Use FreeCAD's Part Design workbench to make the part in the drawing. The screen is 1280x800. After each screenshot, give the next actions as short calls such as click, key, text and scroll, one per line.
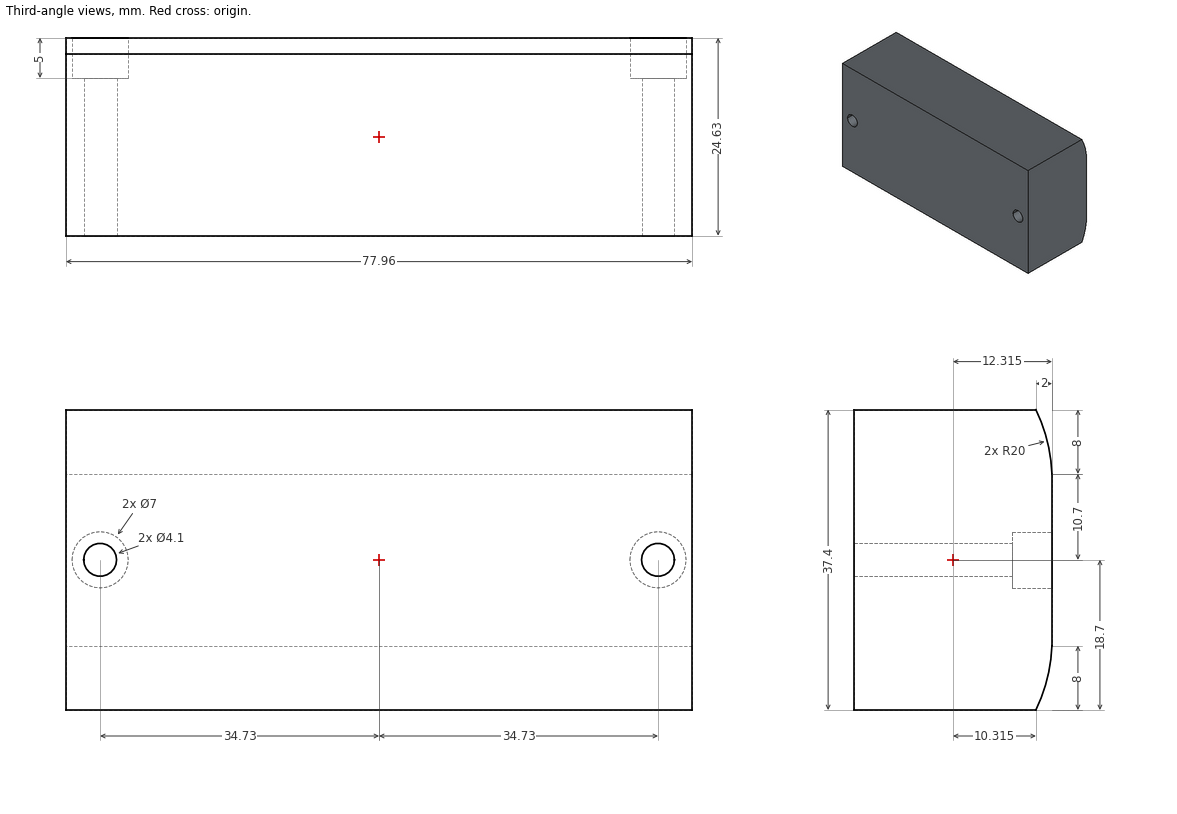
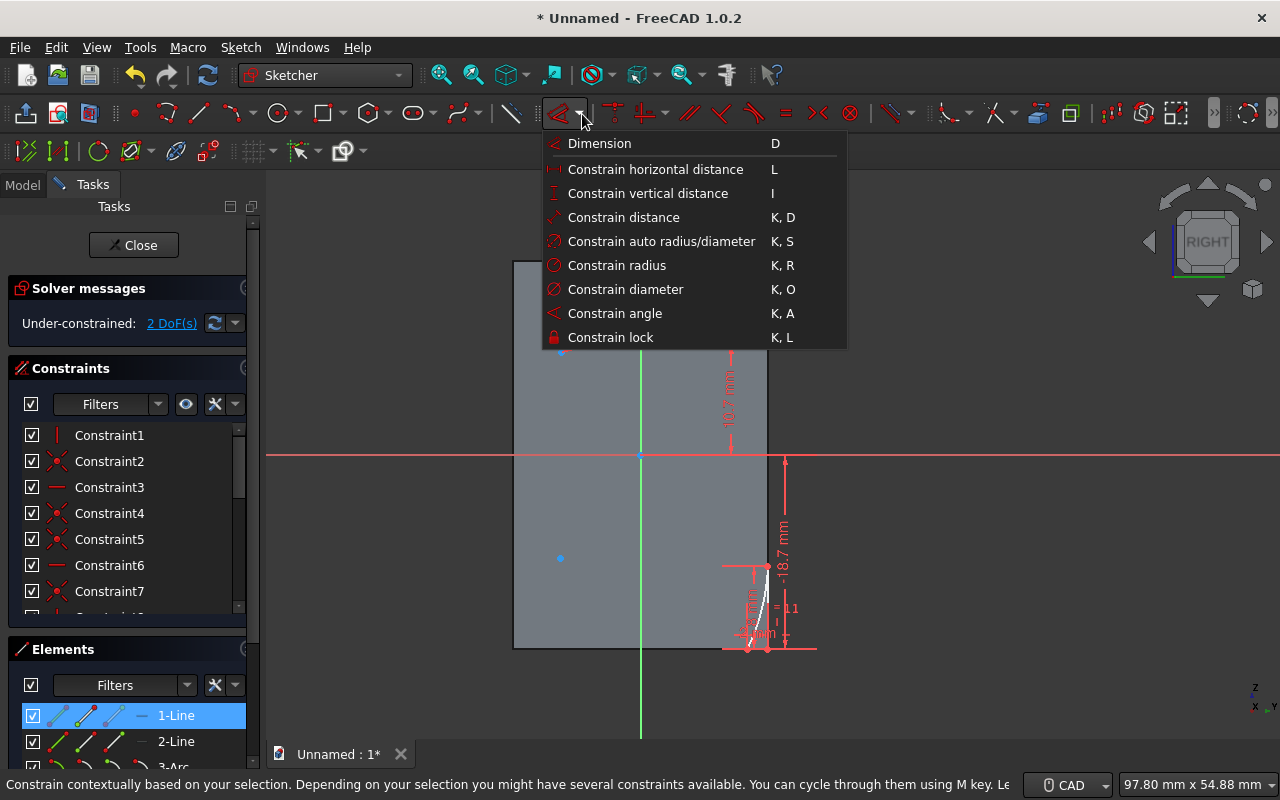
click(695, 169)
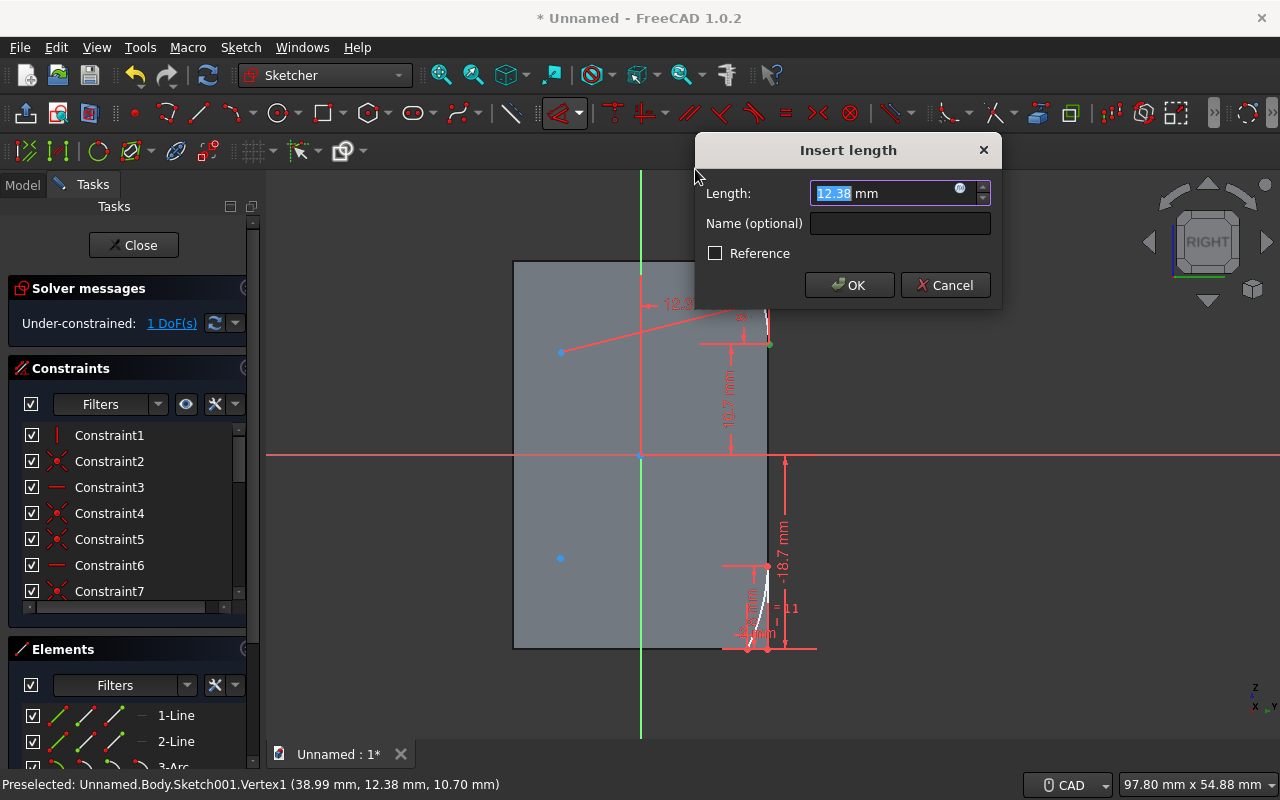
text(12.315)
key(Return)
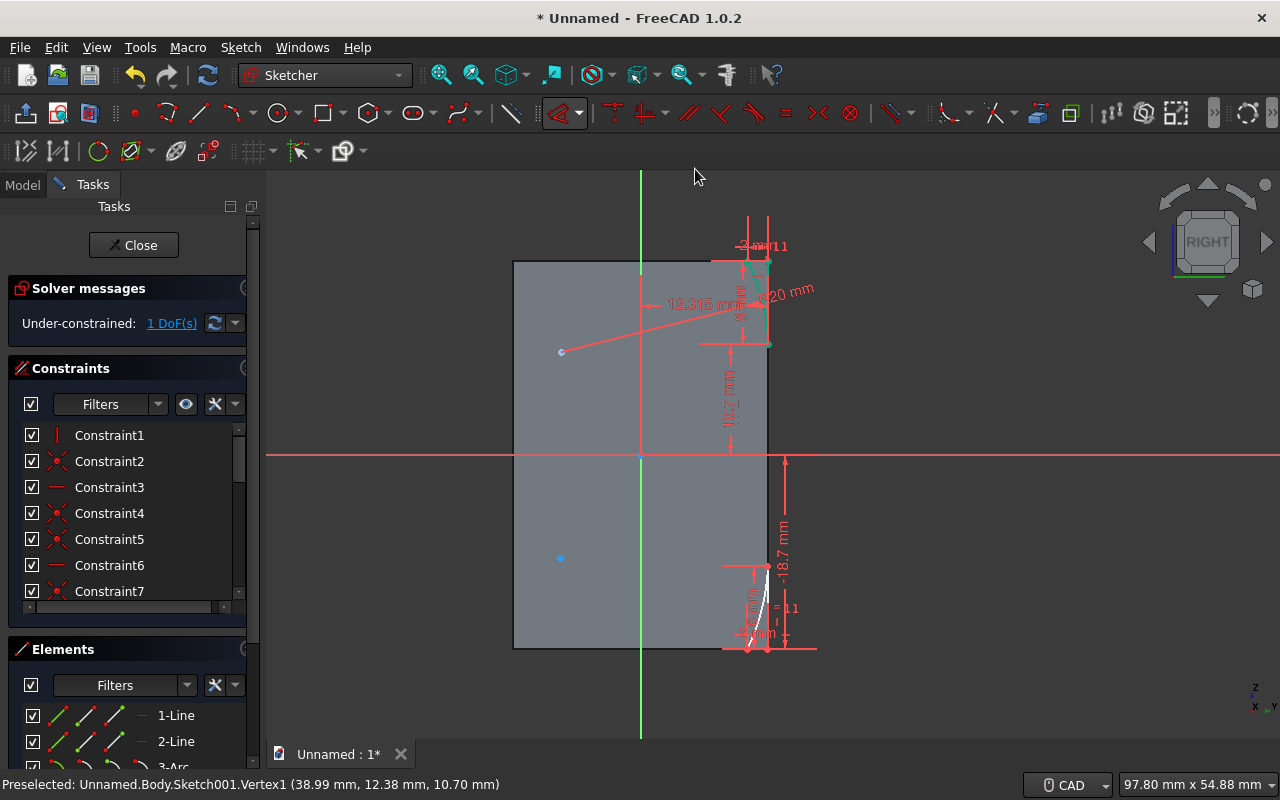
click(747, 649)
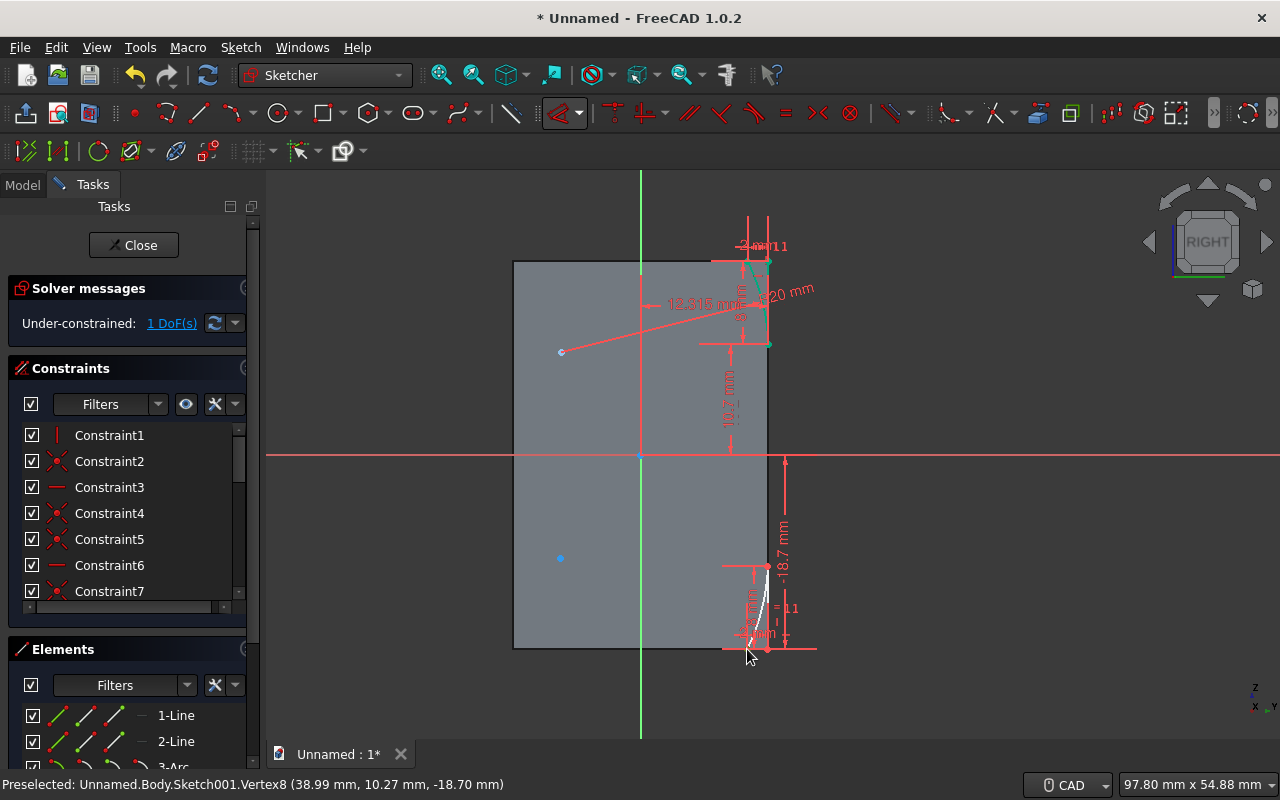
click(582, 114)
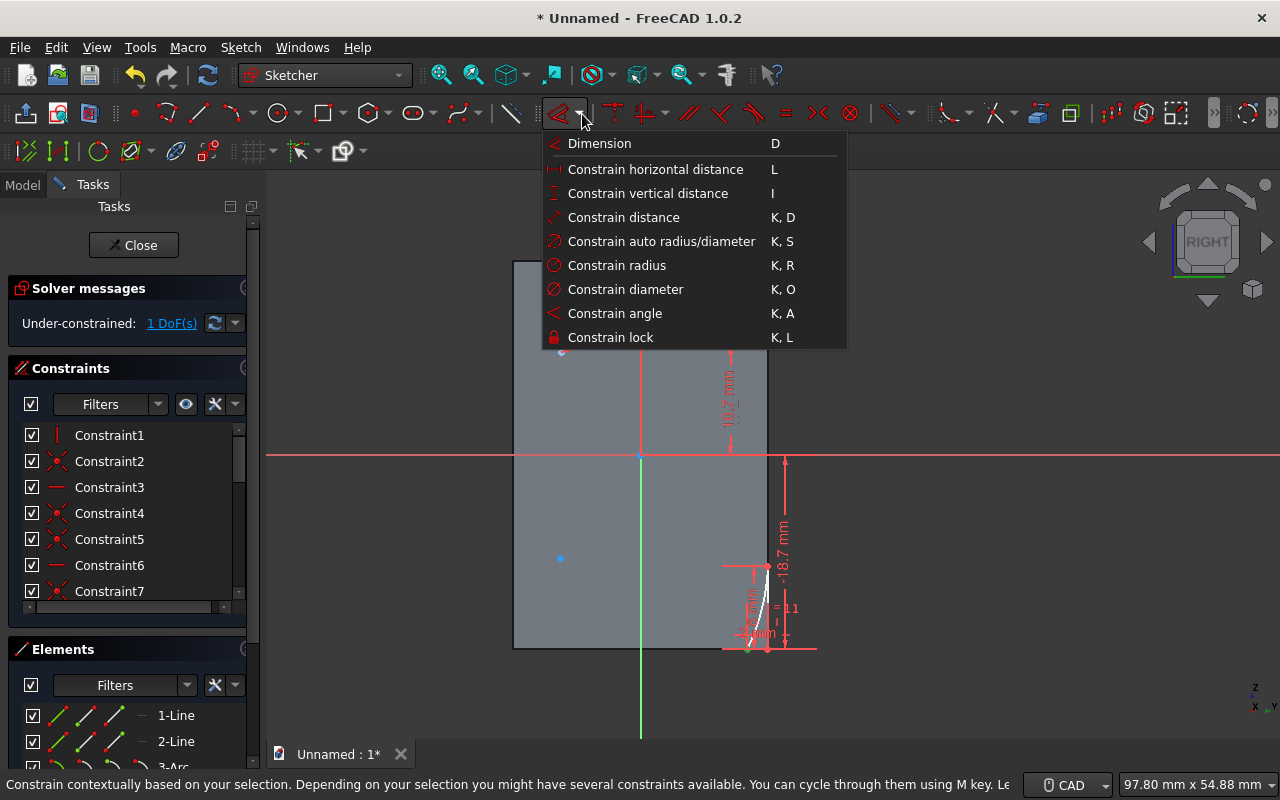
click(695, 169)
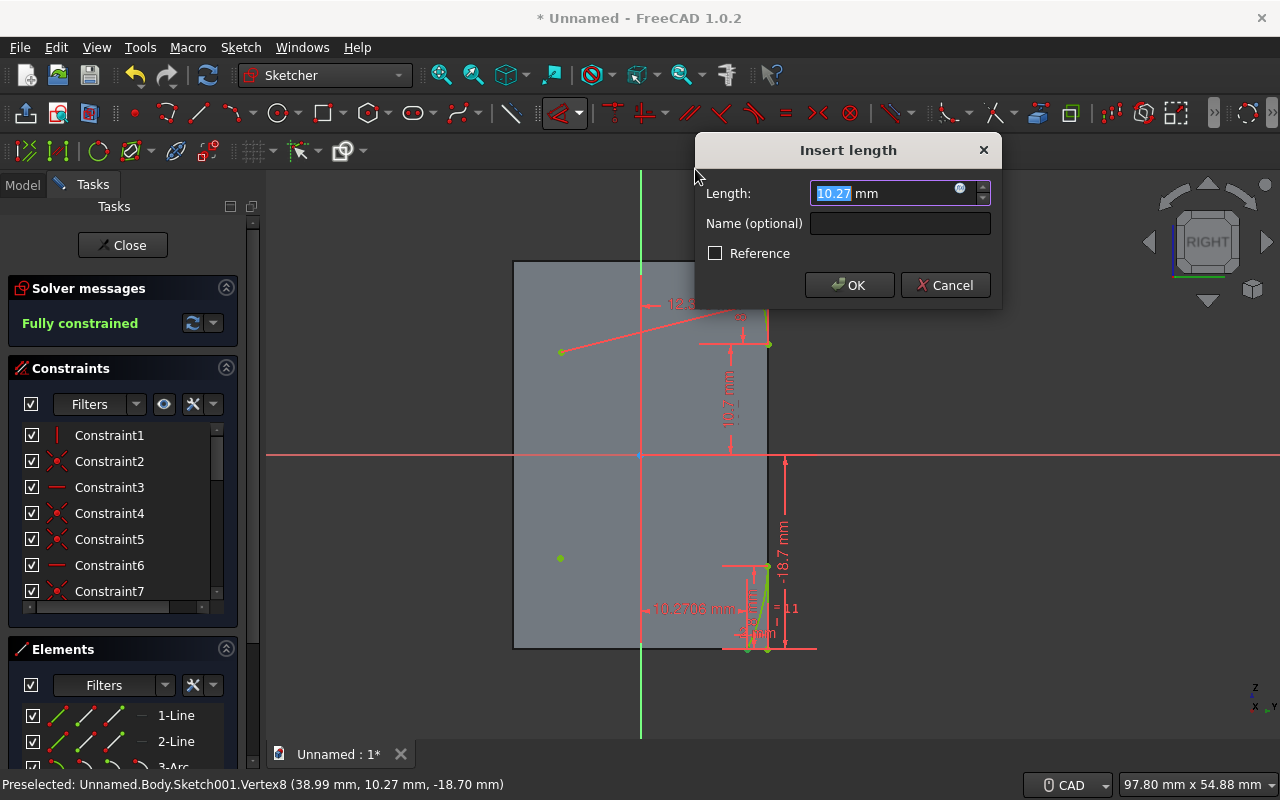
text(10.315)
key(Return)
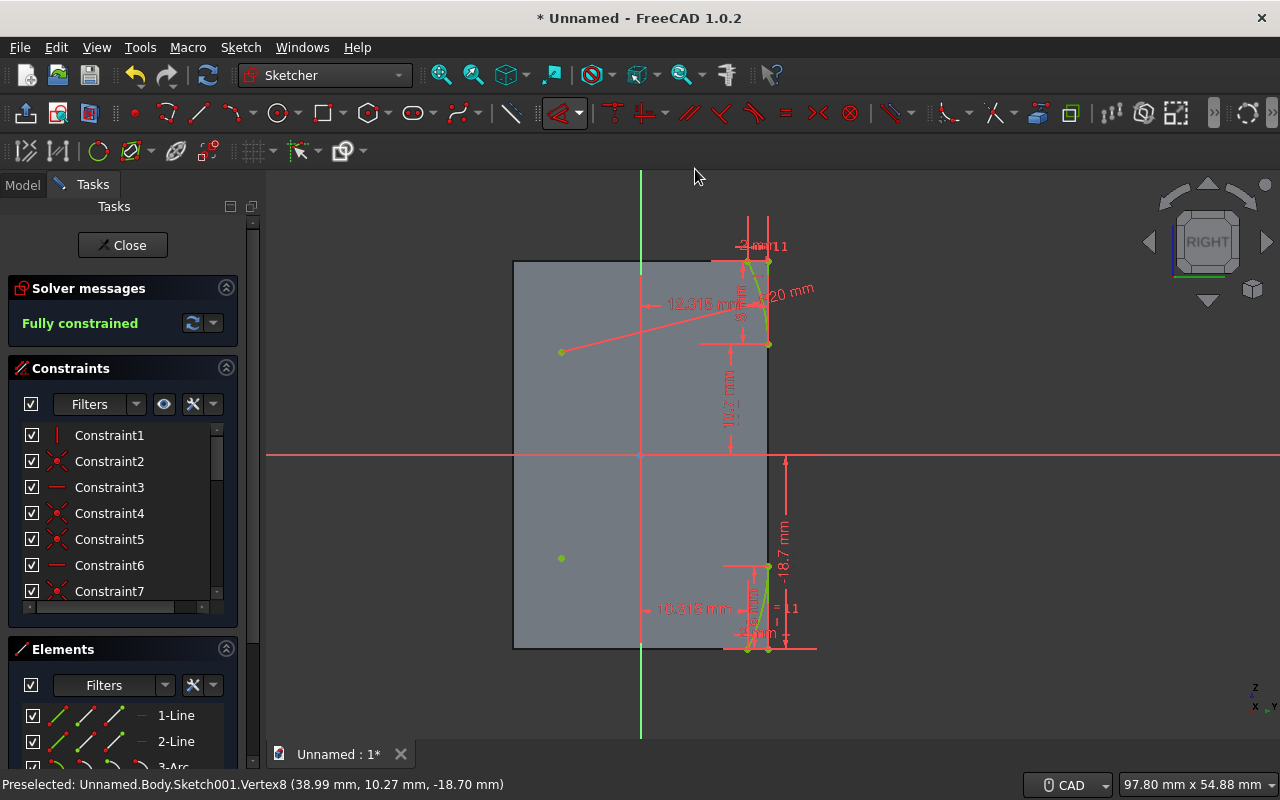
click(123, 245)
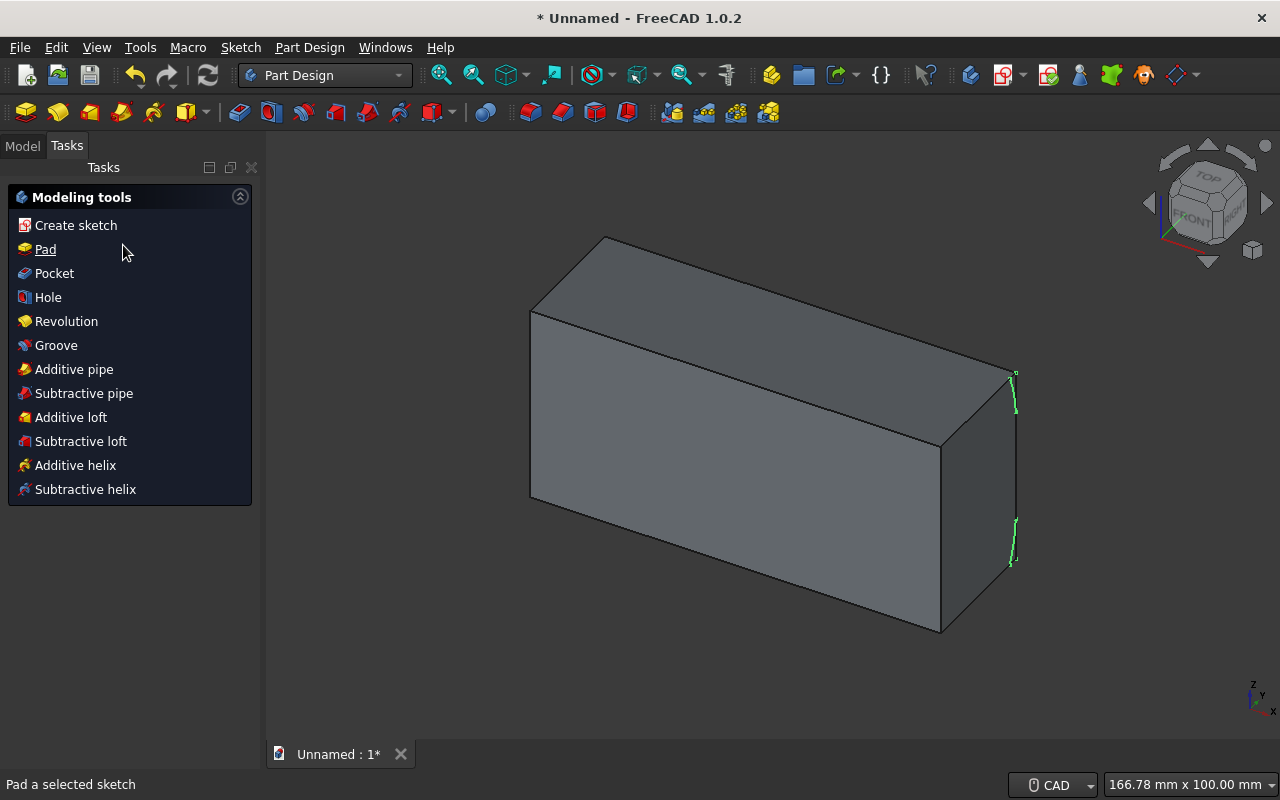
click(240, 112)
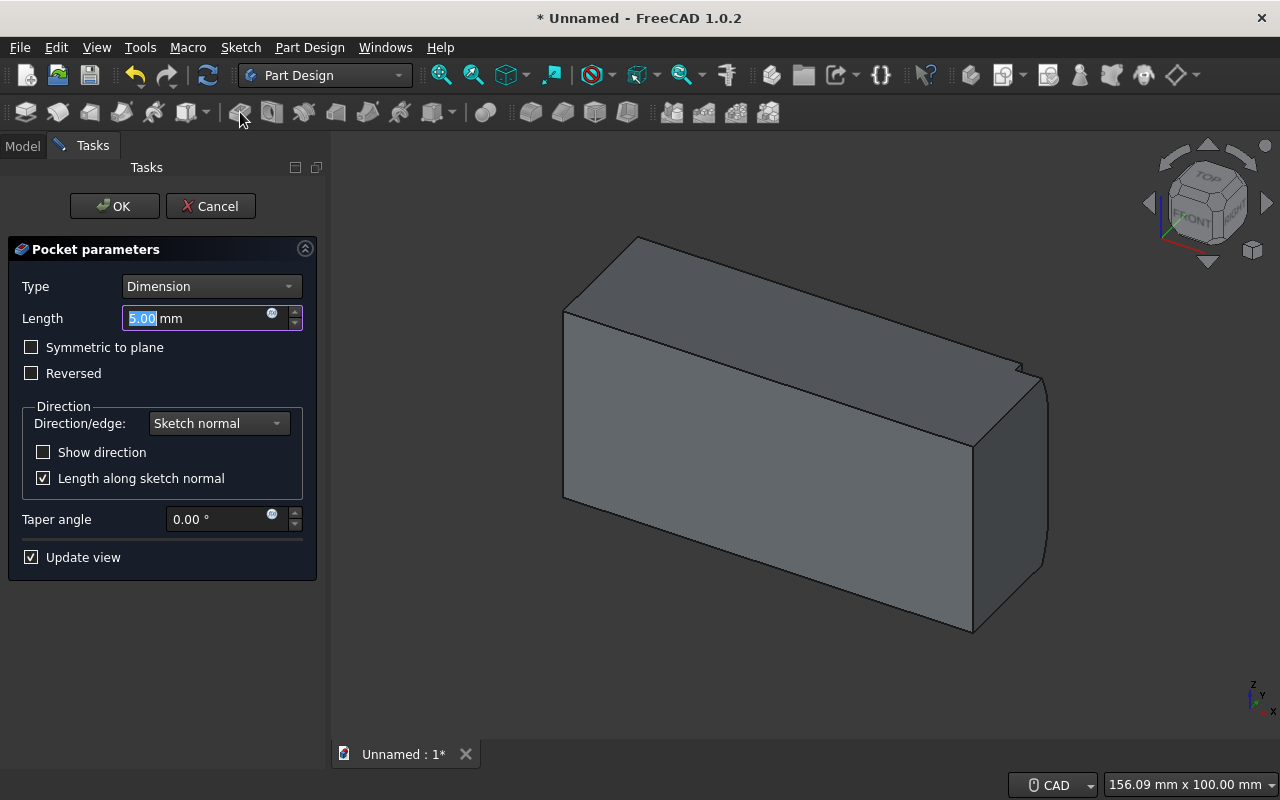
click(212, 286)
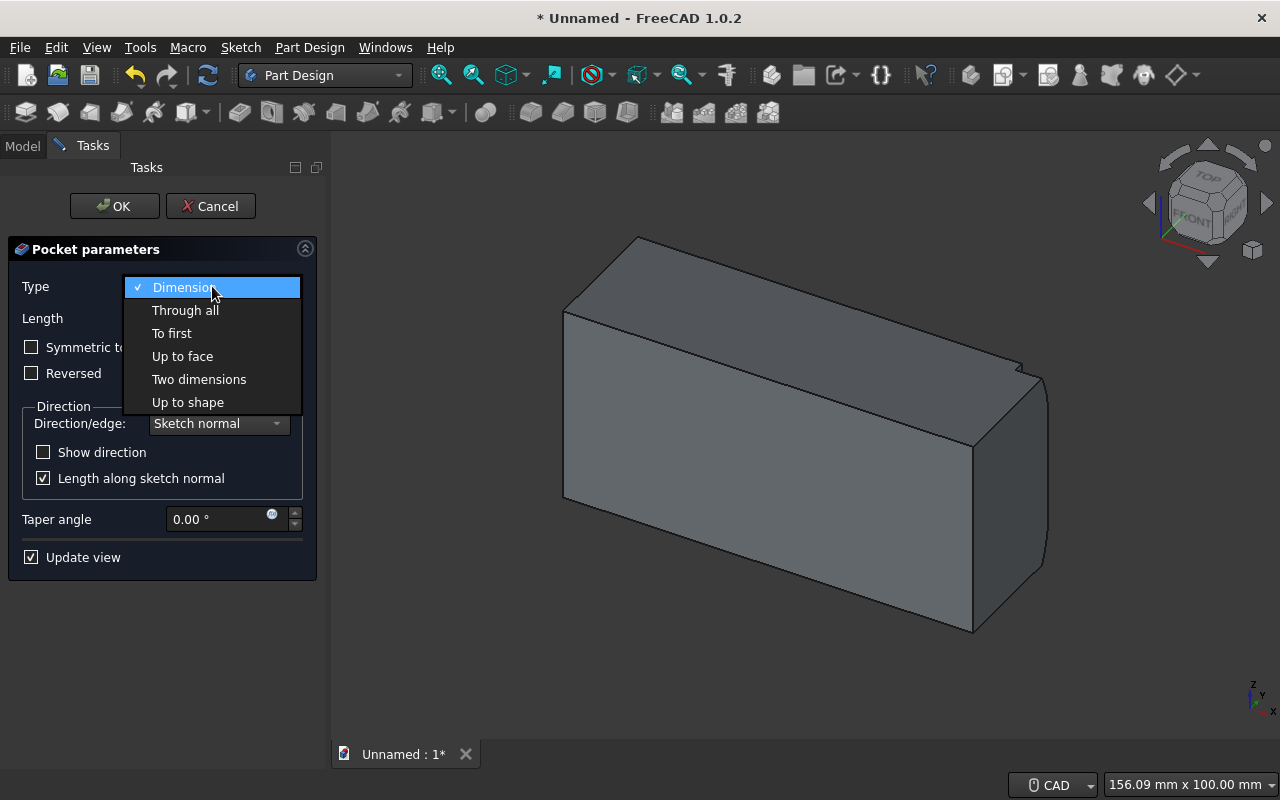
click(212, 310)